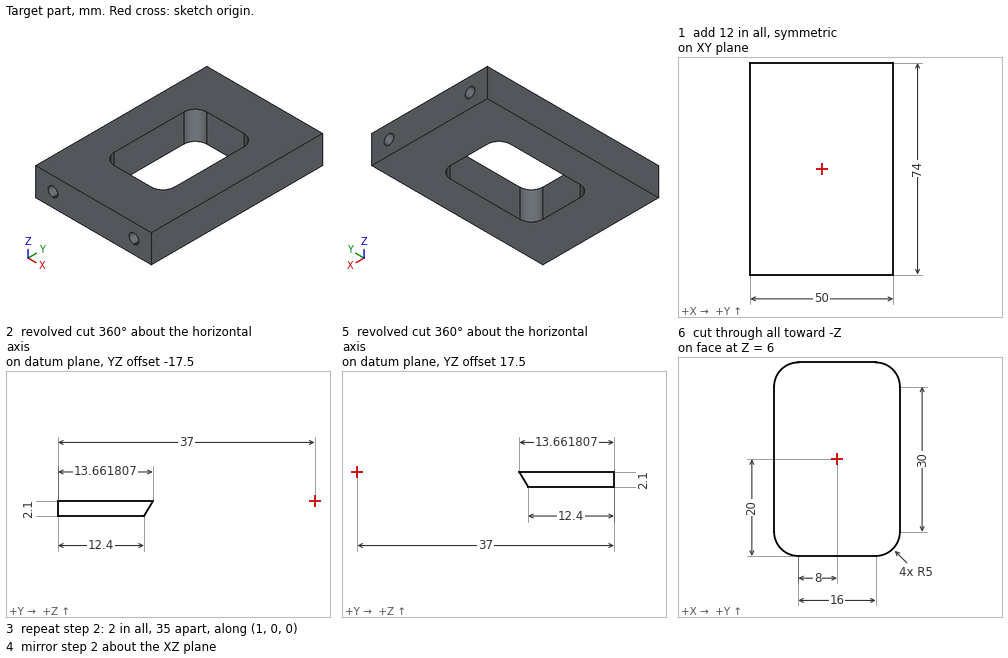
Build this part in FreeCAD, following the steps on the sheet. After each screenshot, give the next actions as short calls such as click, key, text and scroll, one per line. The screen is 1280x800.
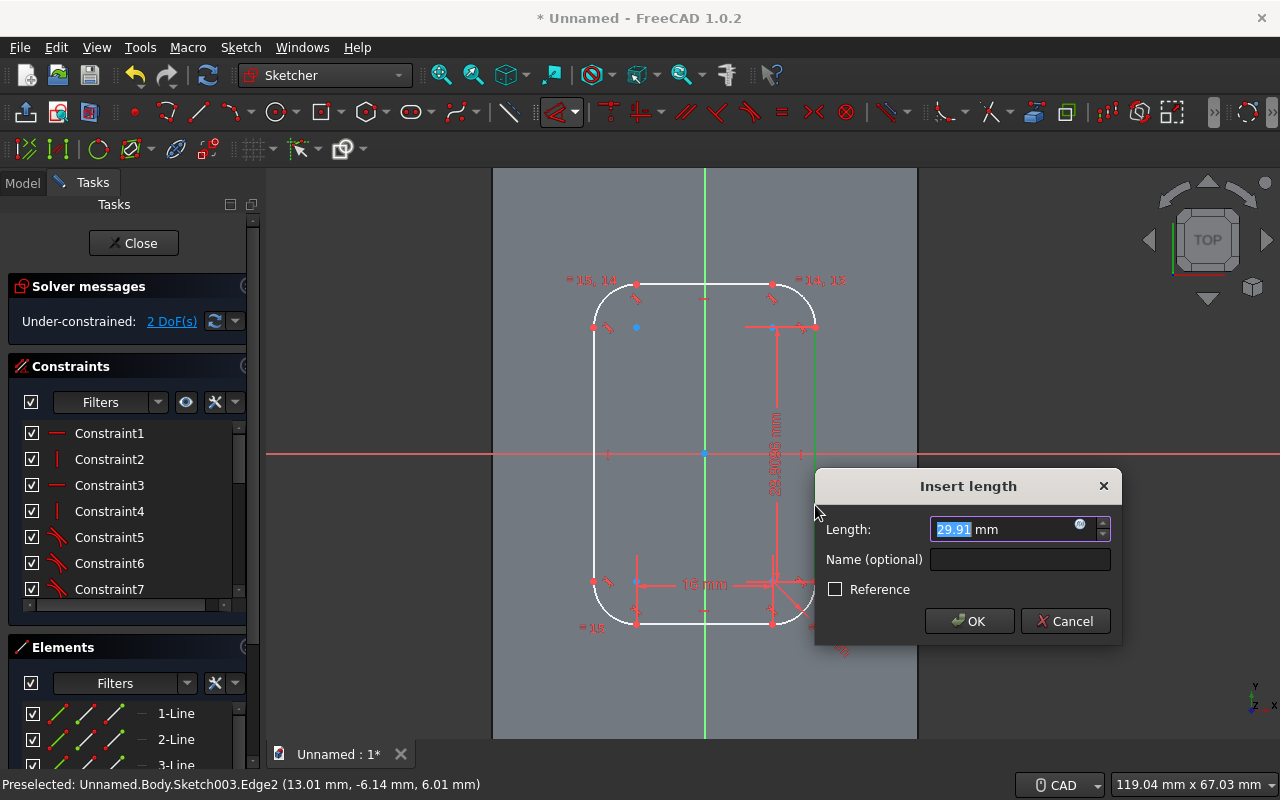
text(30)
key(Return)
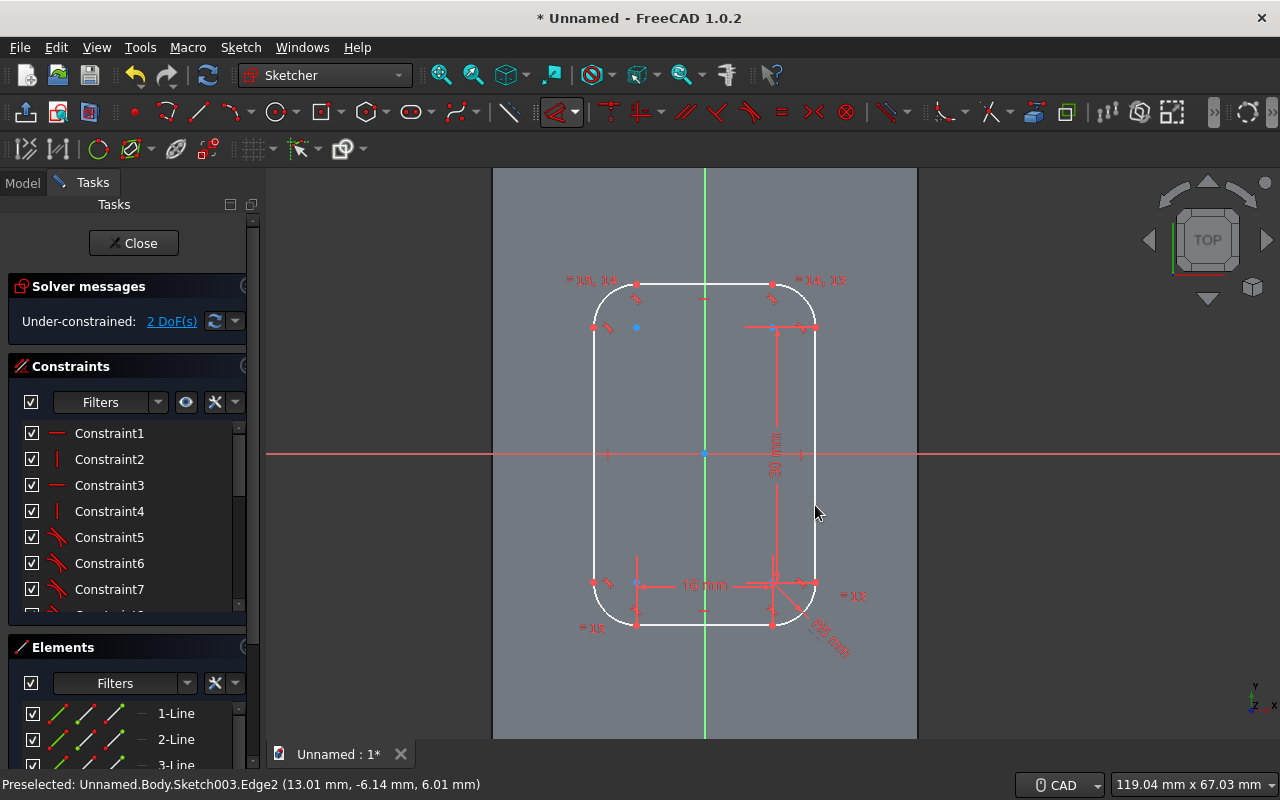
click(637, 625)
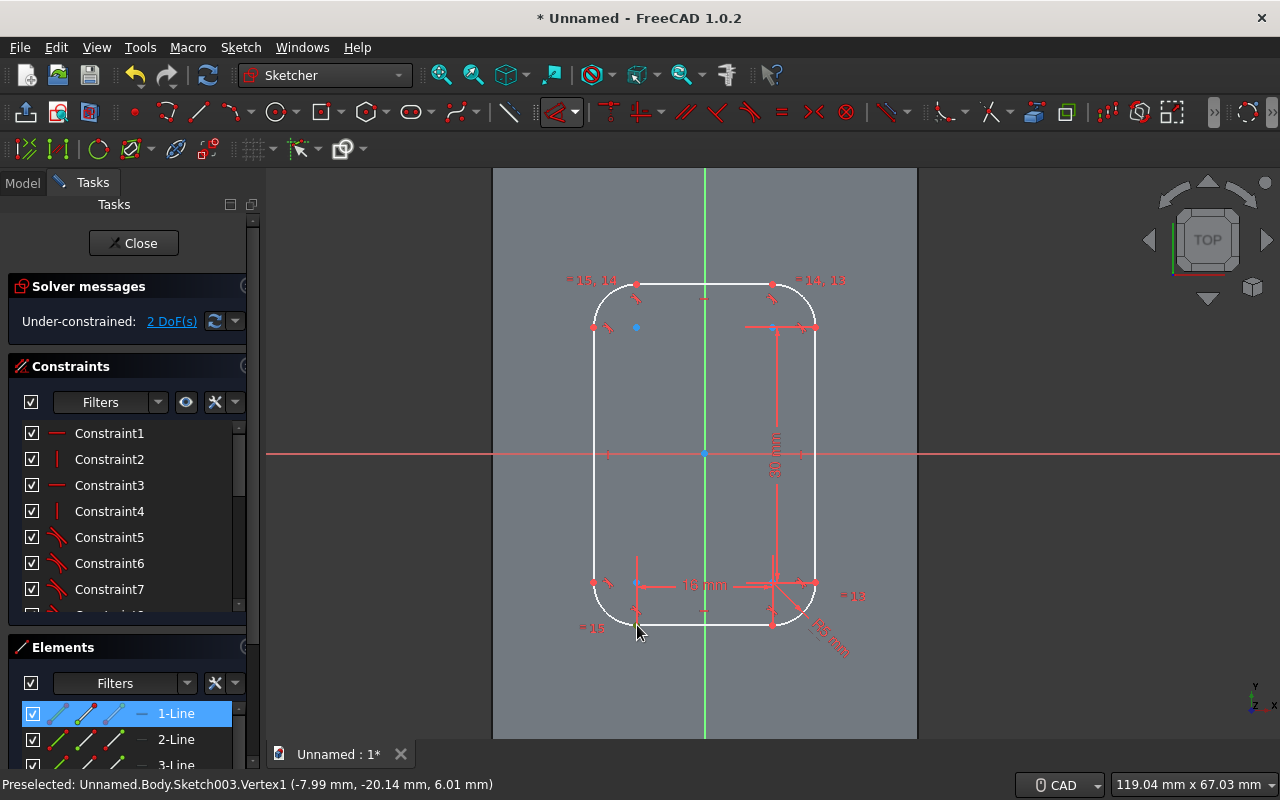
key(l)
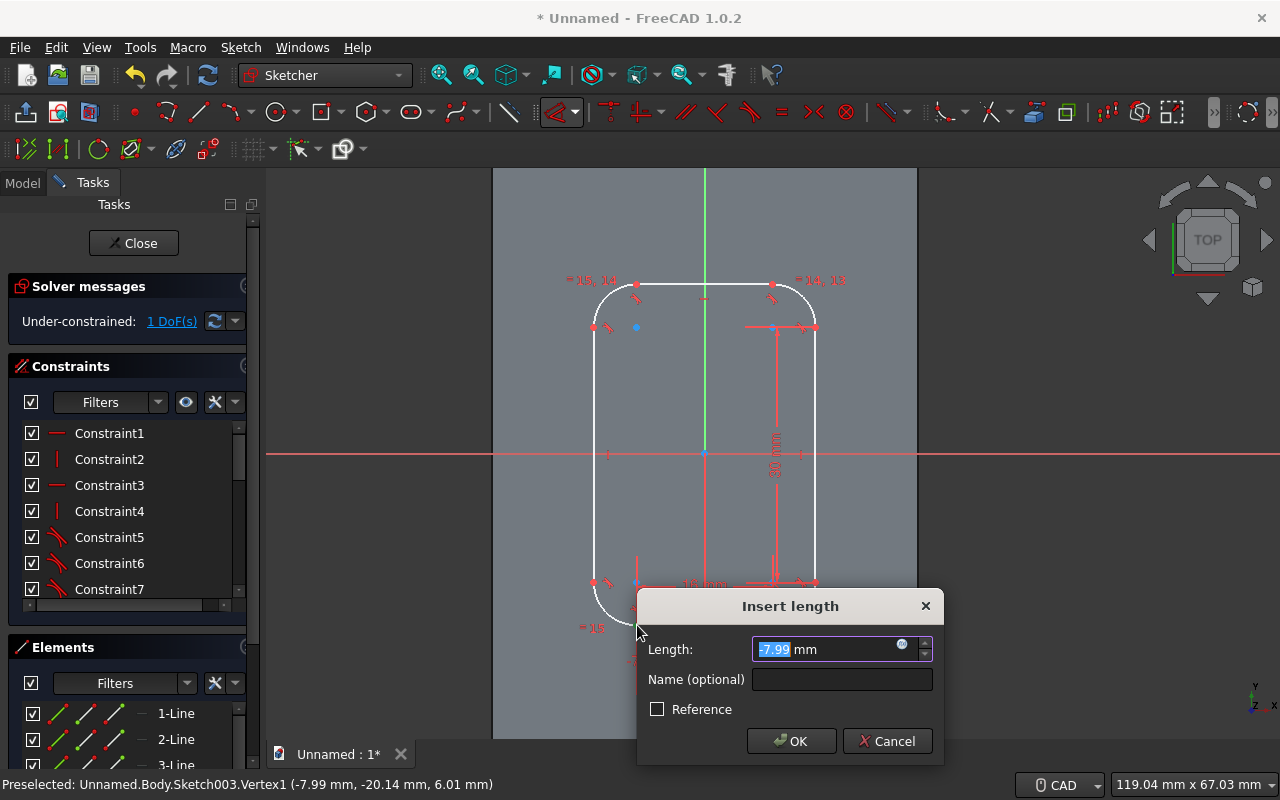
text(-8)
key(Return)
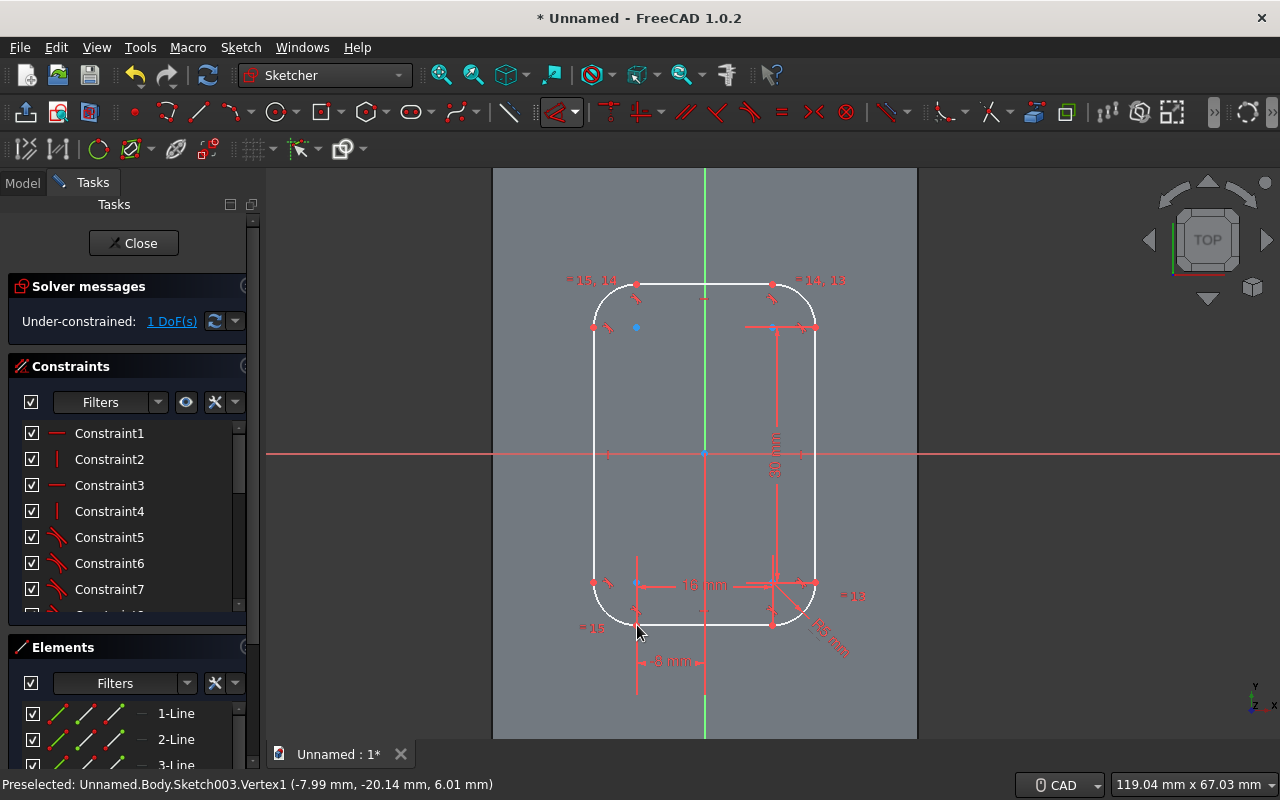
click(637, 625)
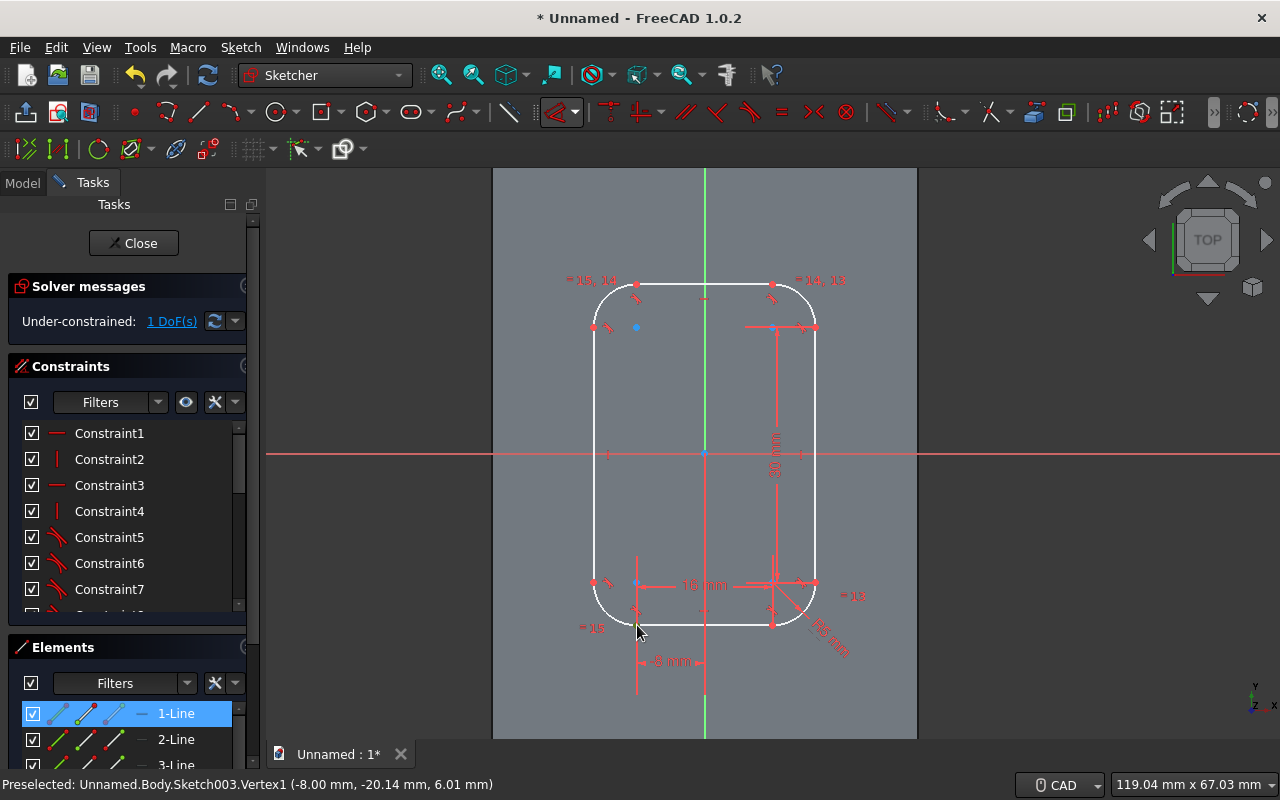
click(578, 112)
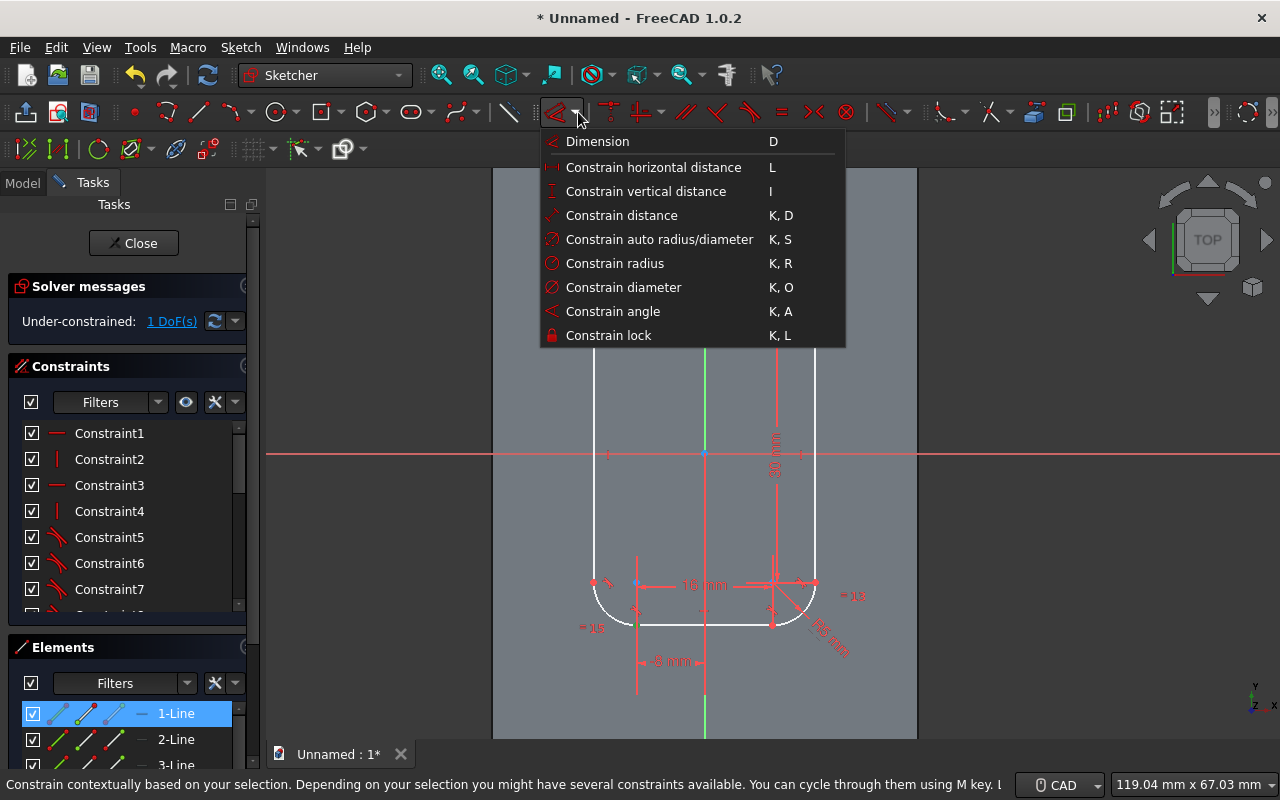
click(693, 191)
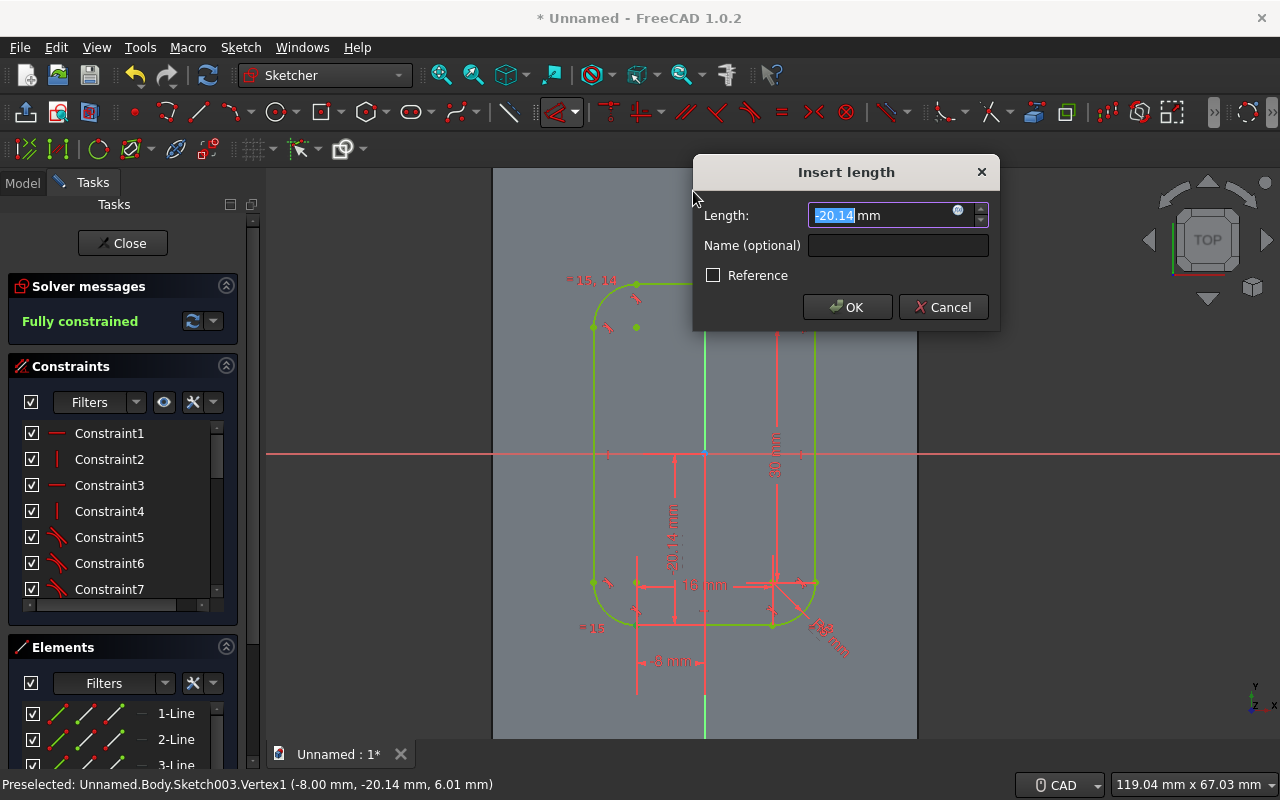
text(-20)
key(Return)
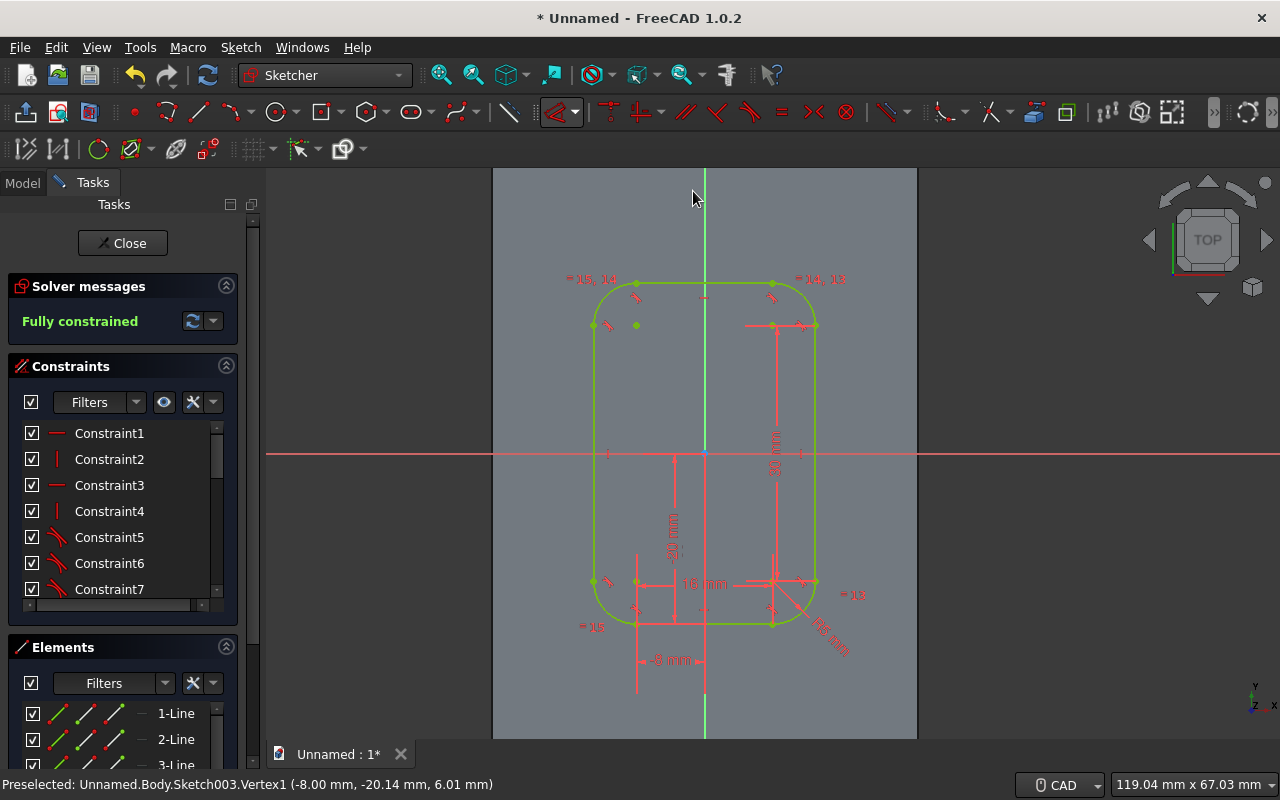
click(123, 243)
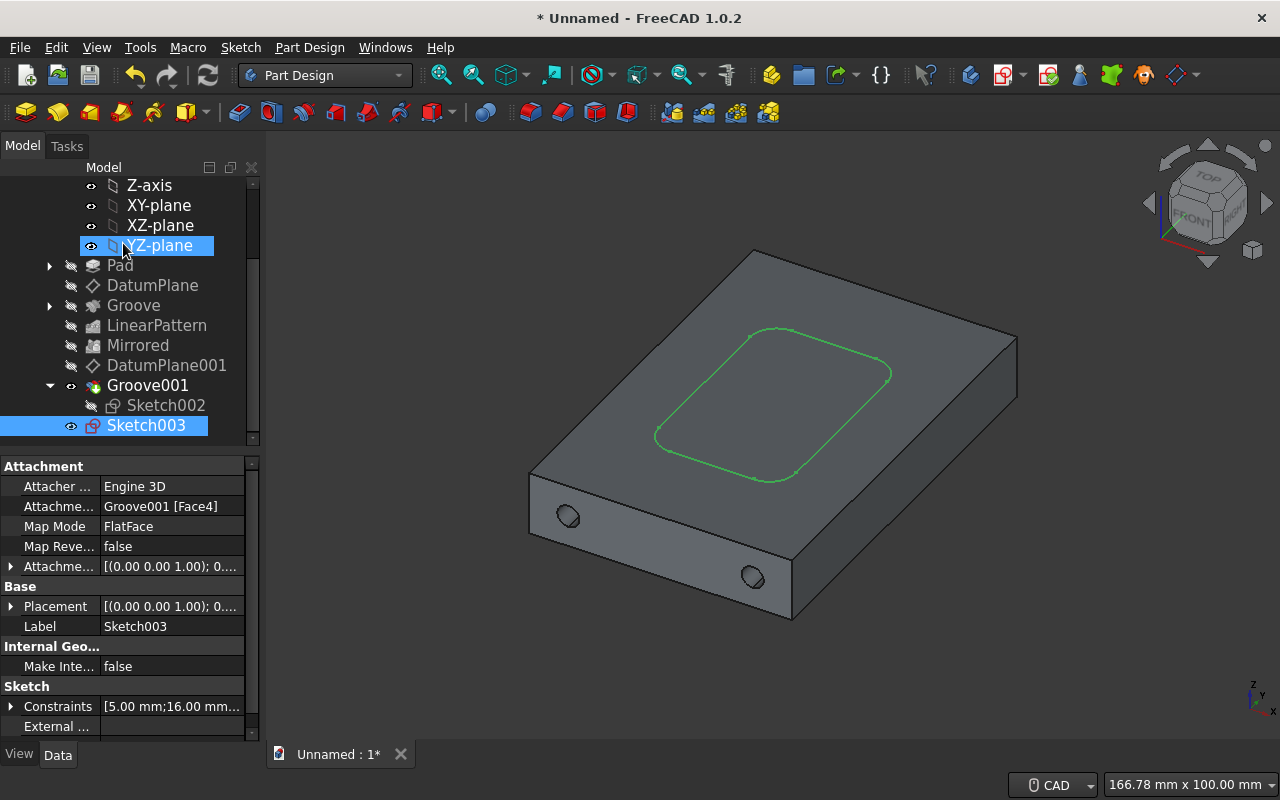
click(240, 112)